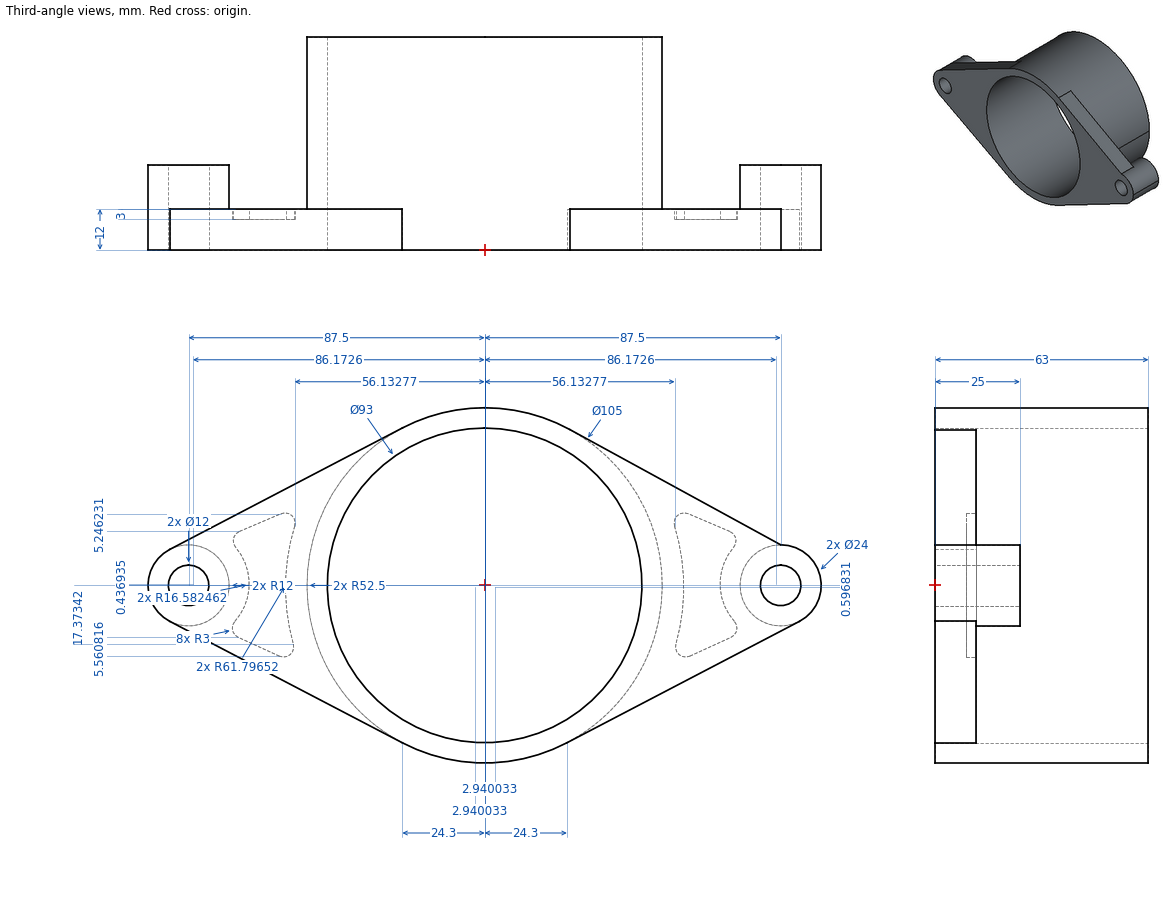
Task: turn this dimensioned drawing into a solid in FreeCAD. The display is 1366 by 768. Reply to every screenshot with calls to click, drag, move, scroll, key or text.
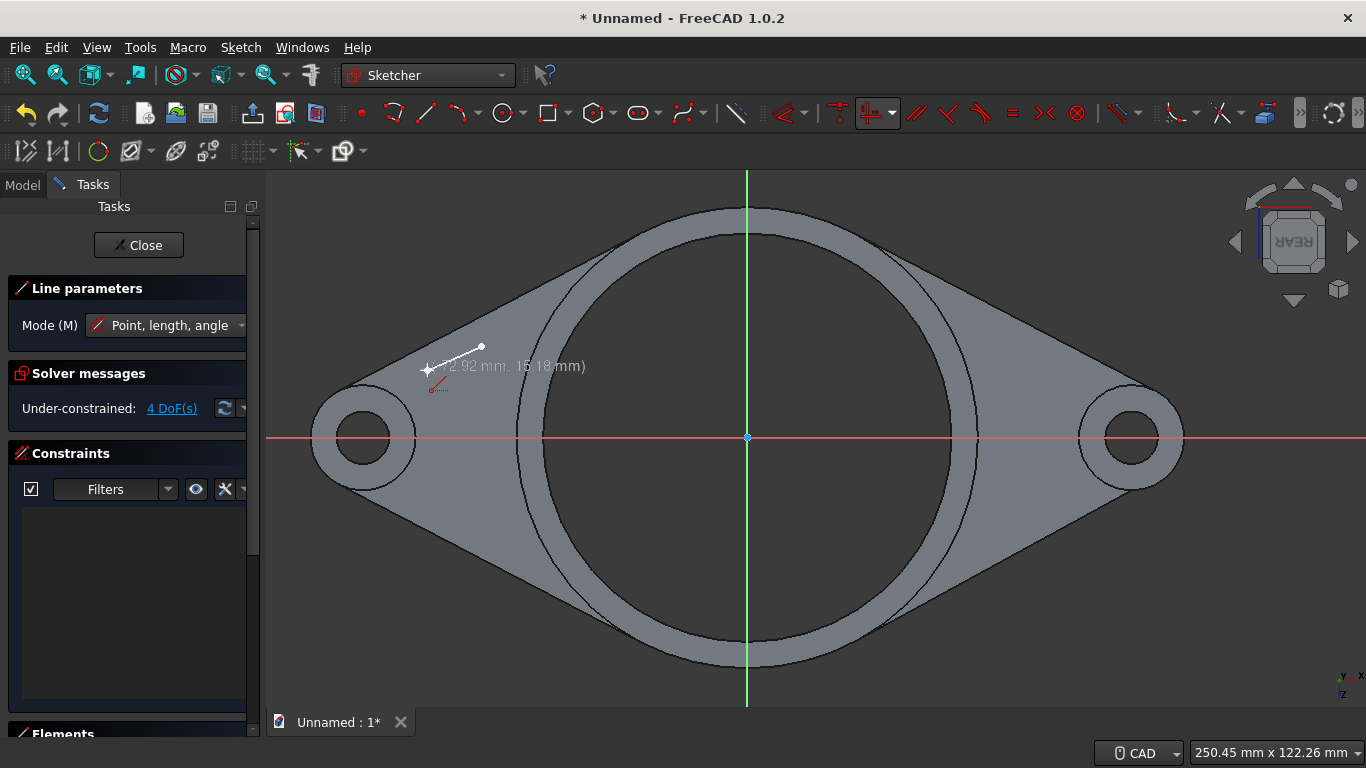
click(429, 508)
click(483, 531)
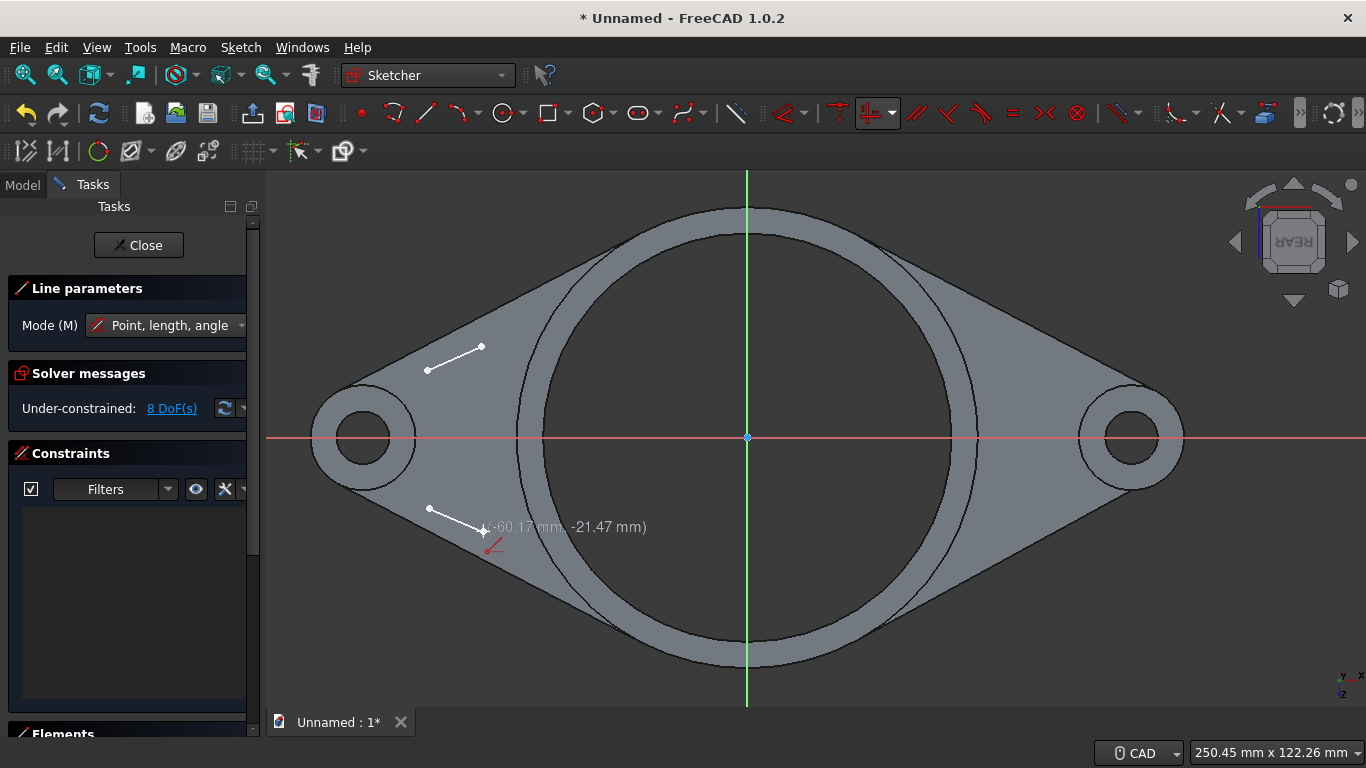
click(458, 114)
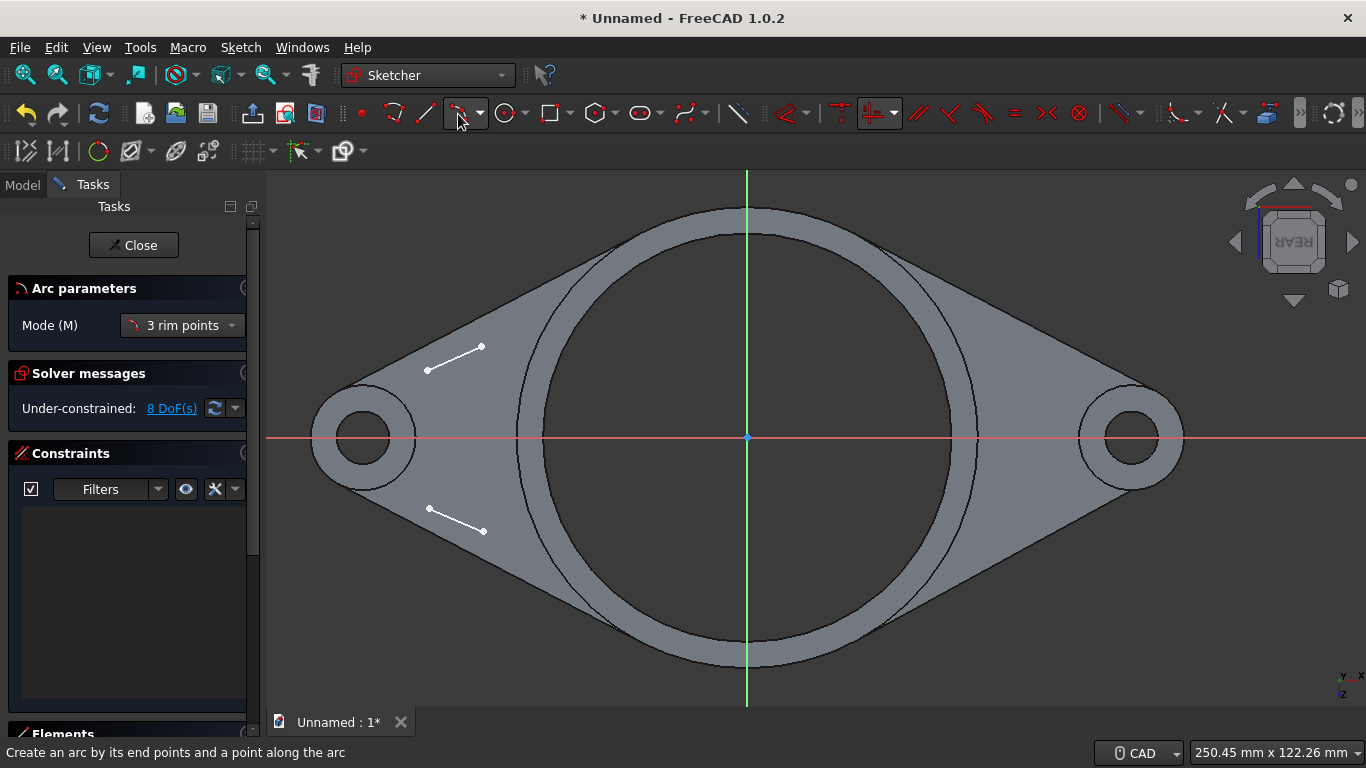
click(427, 371)
click(423, 391)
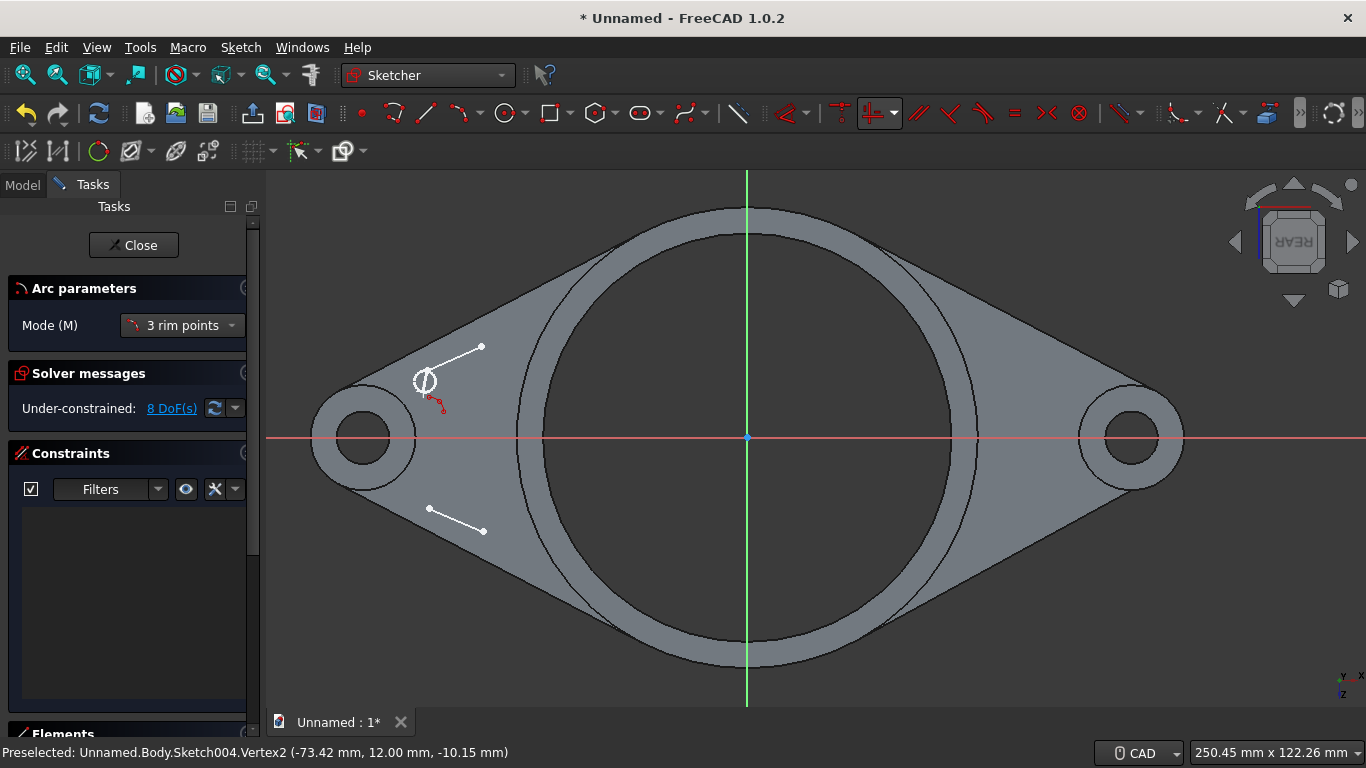
scroll(420, 380, up, 6)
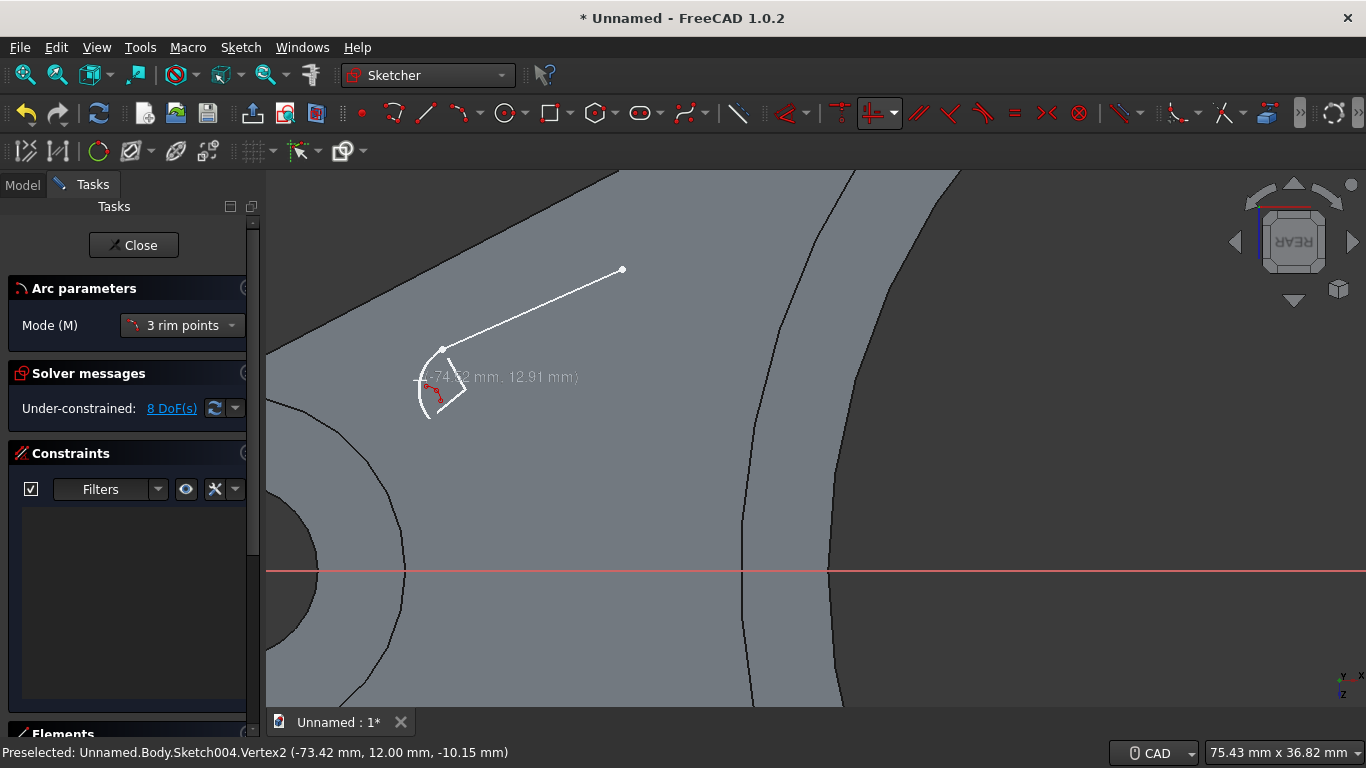
click(420, 378)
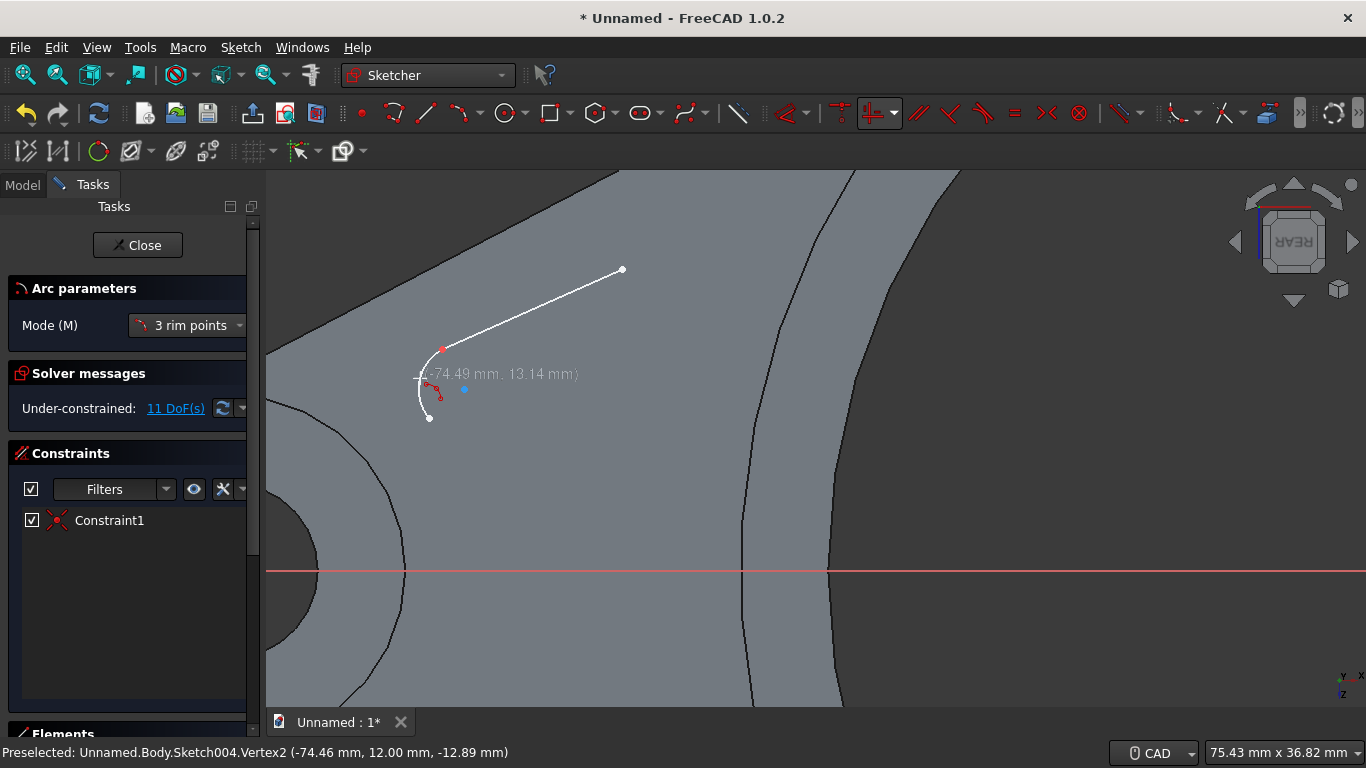
click(430, 419)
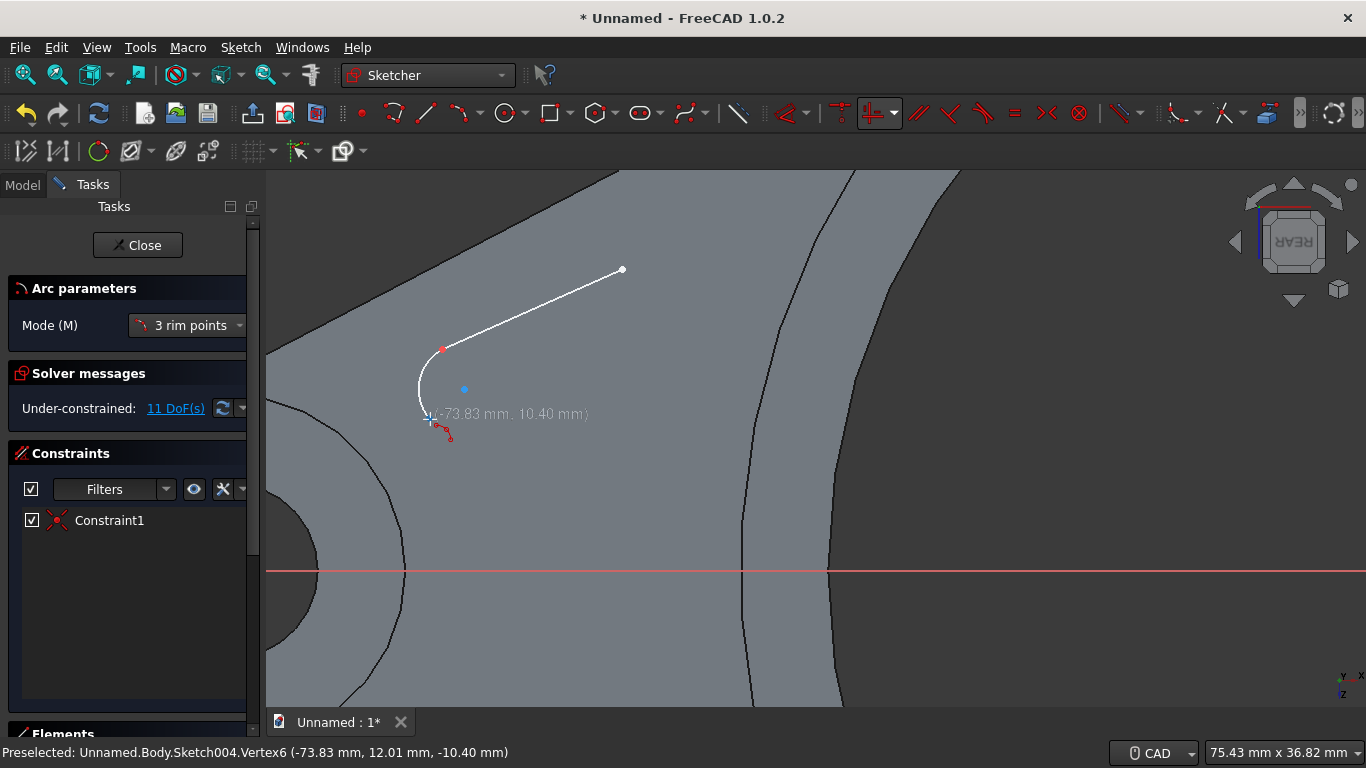
scroll(420, 381, down, 6)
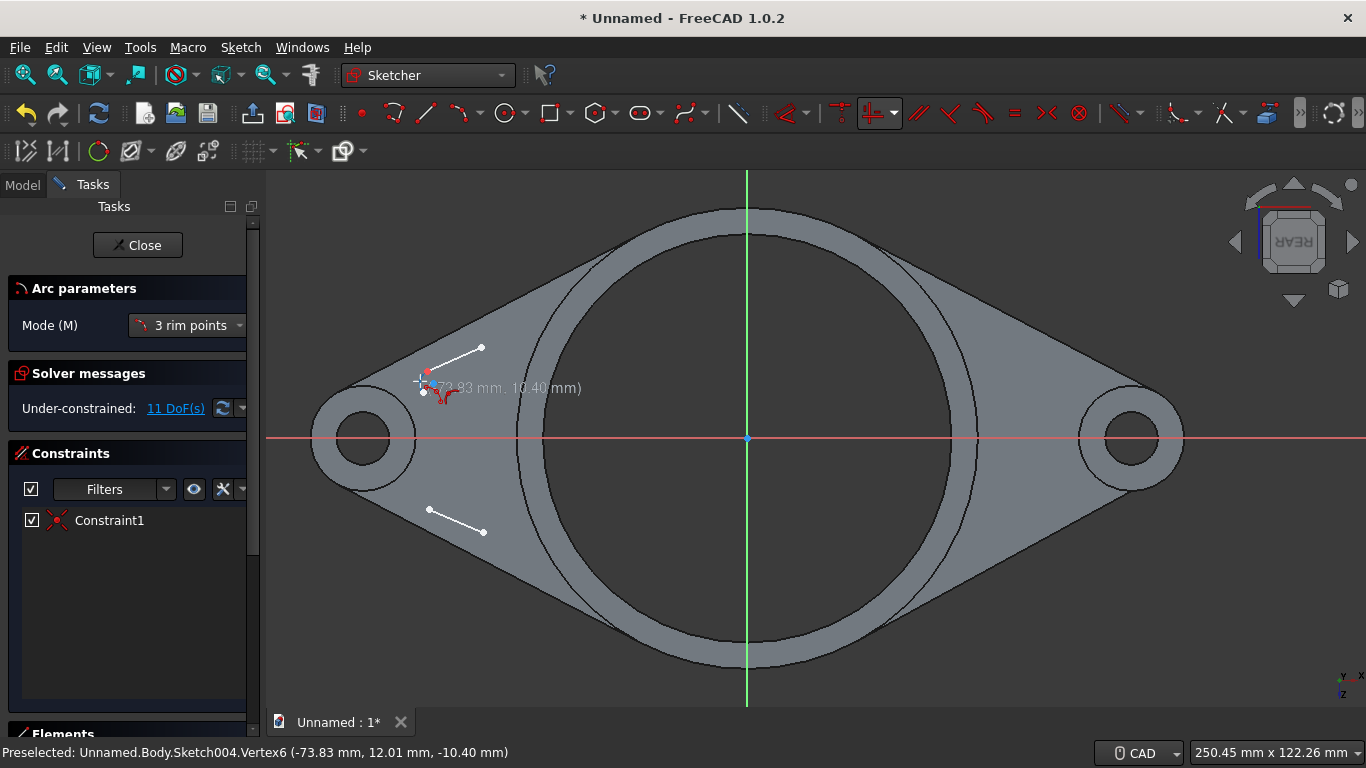
click(424, 488)
click(439, 460)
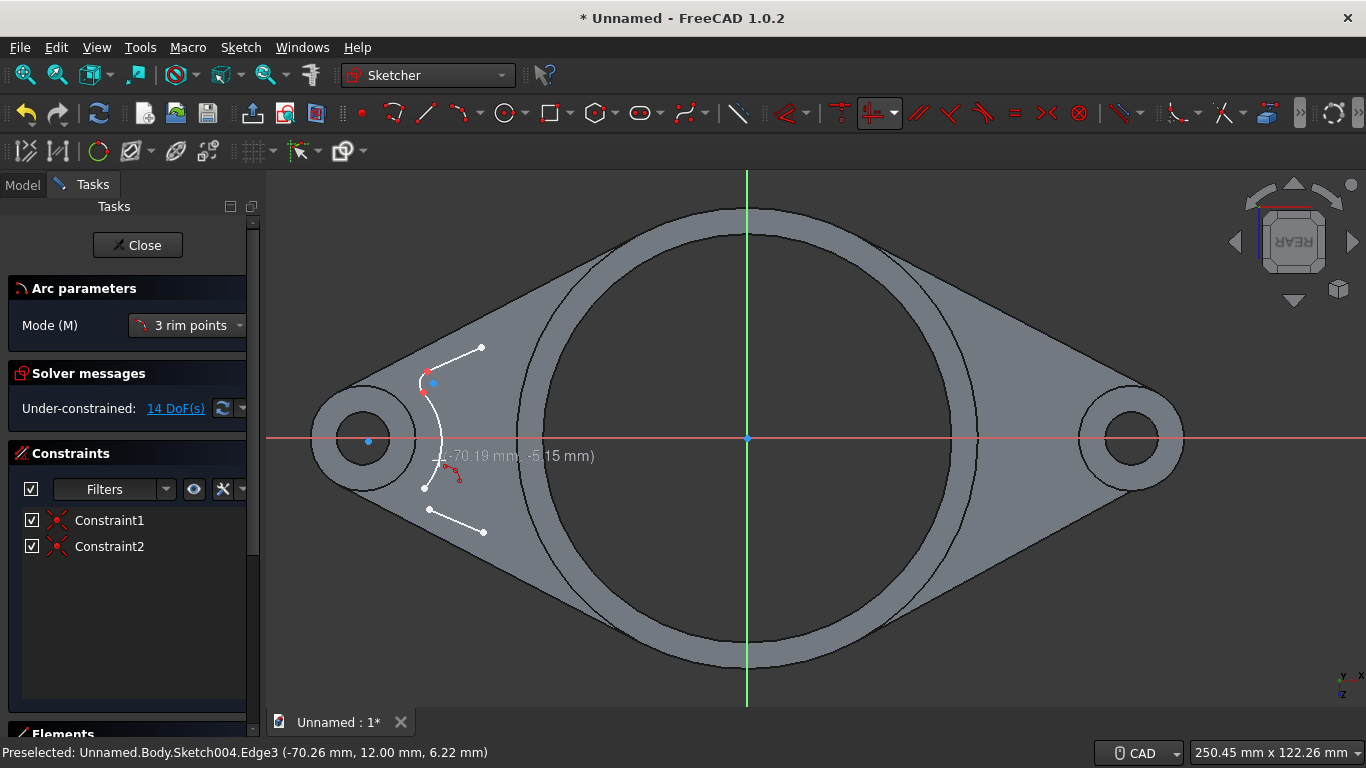
click(424, 489)
click(429, 510)